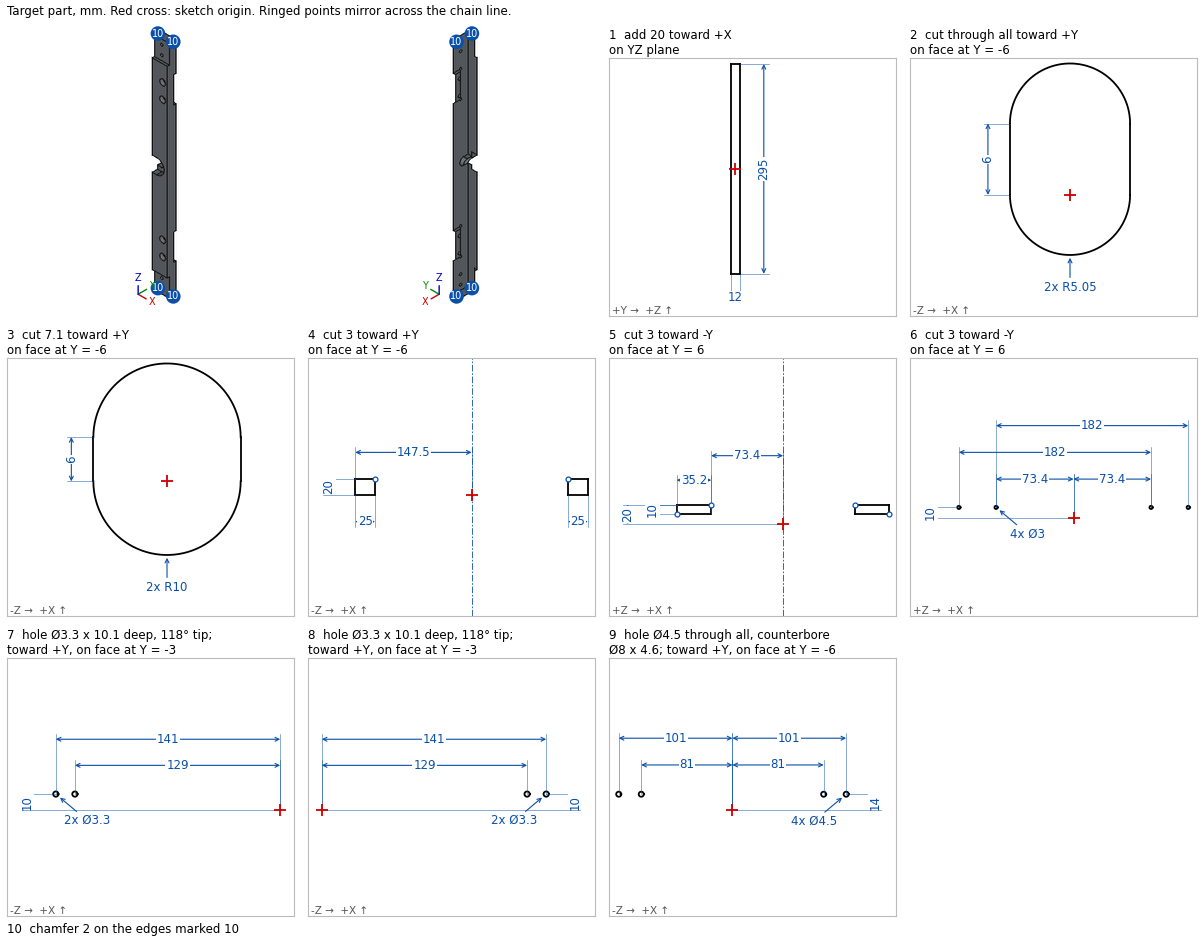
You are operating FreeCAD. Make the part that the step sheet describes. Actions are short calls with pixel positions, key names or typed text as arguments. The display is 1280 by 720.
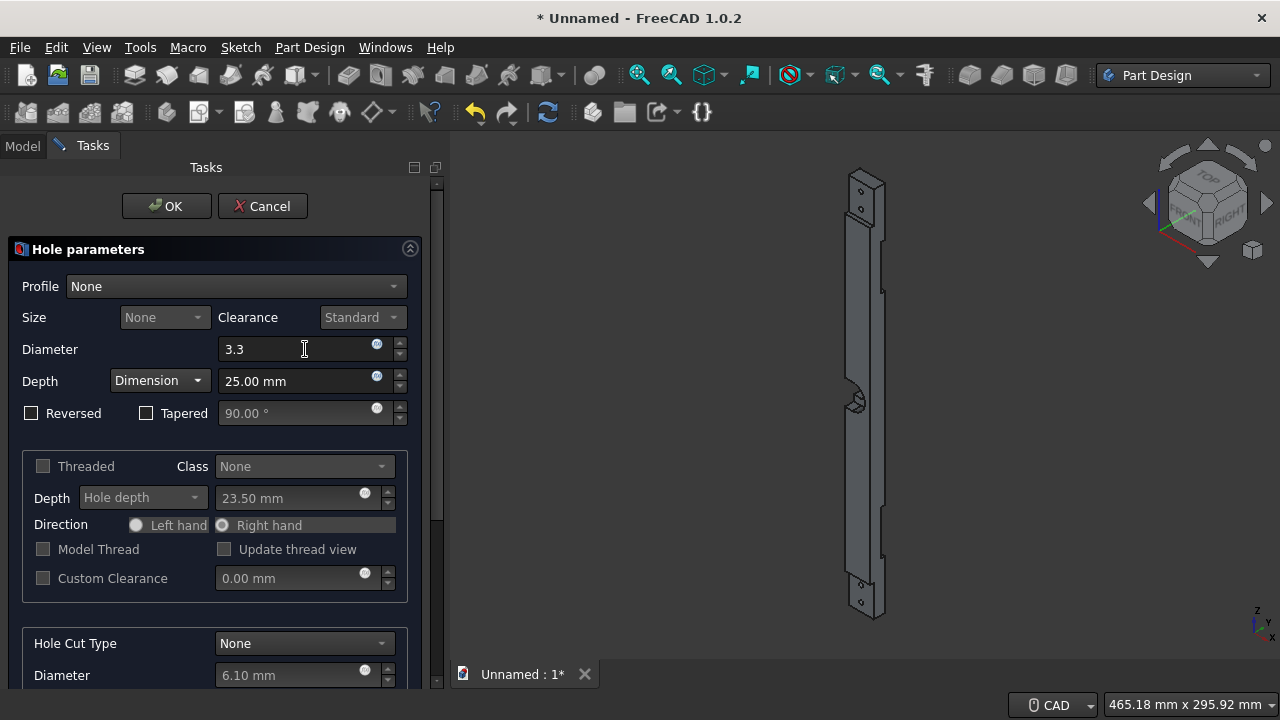
triple_click(305, 381)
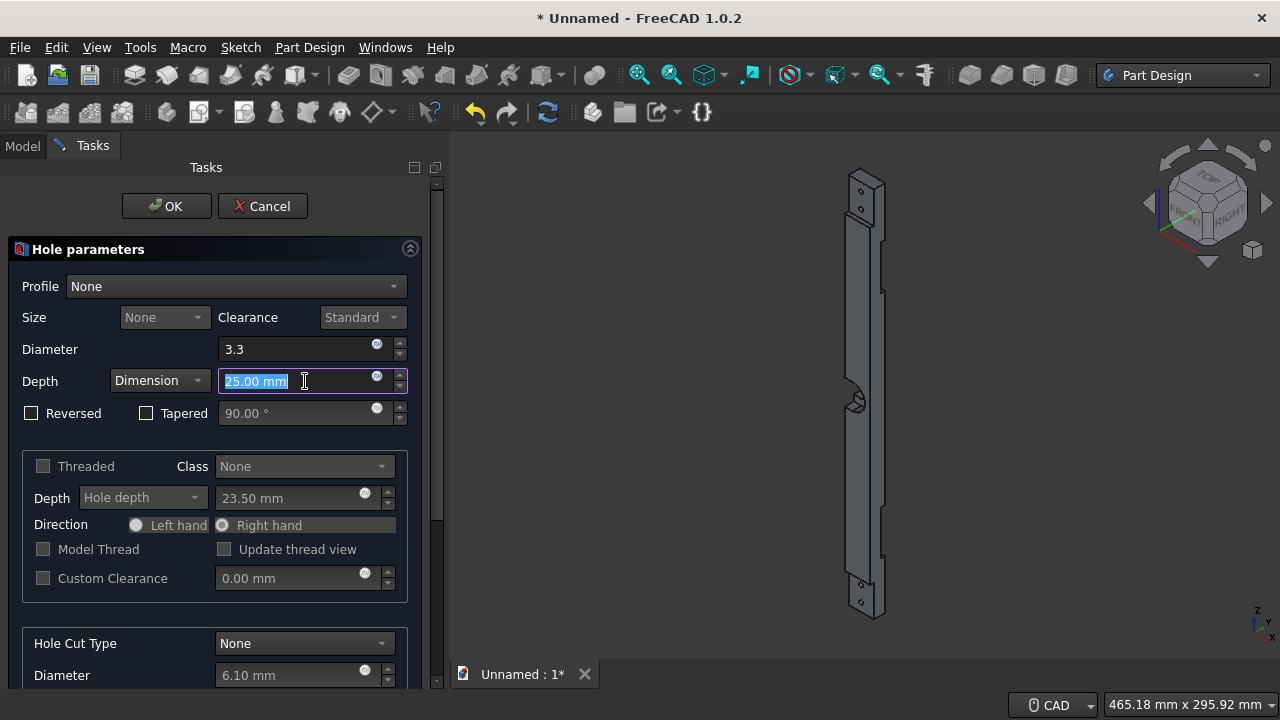
text(10.1)
key(Tab)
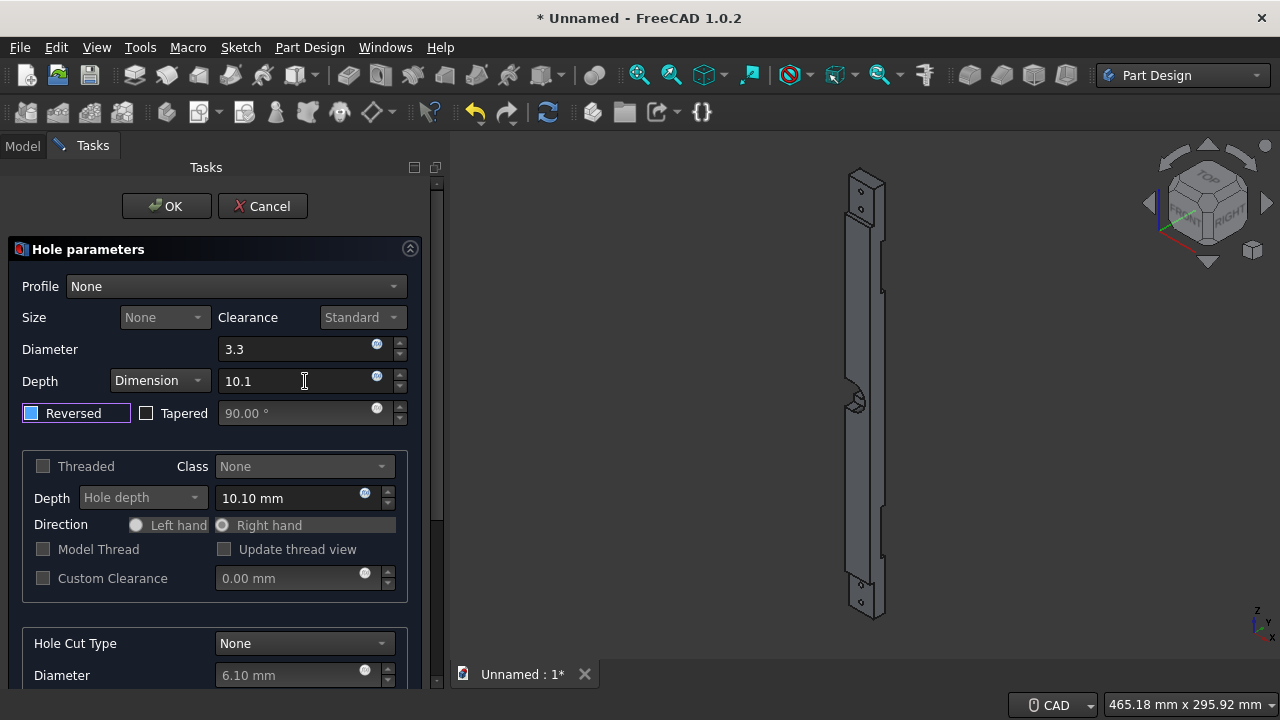
click(167, 206)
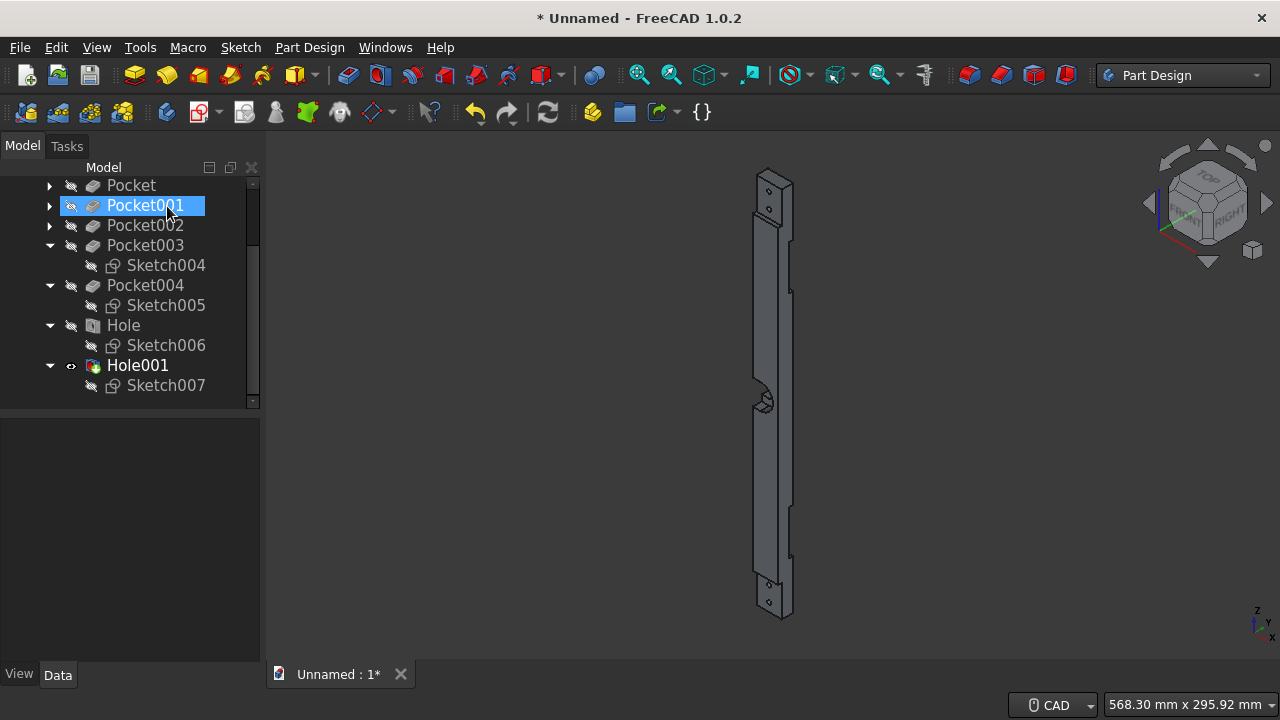
click(765, 347)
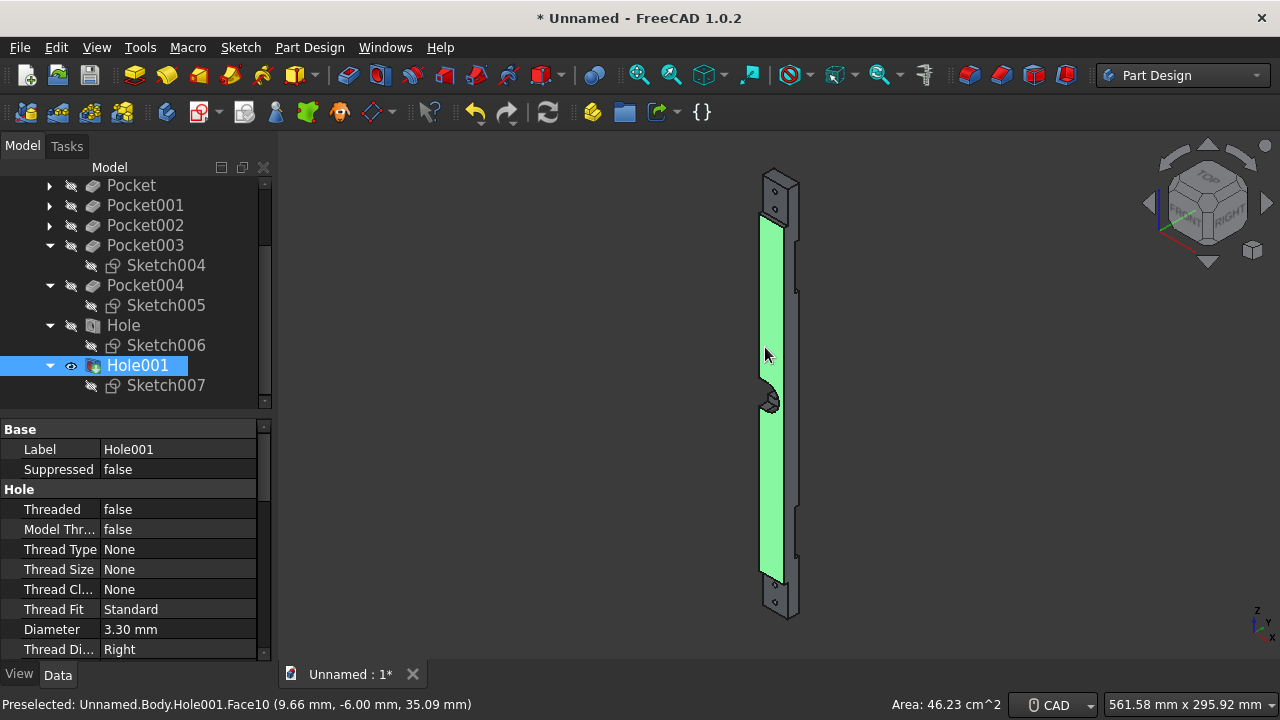
click(200, 112)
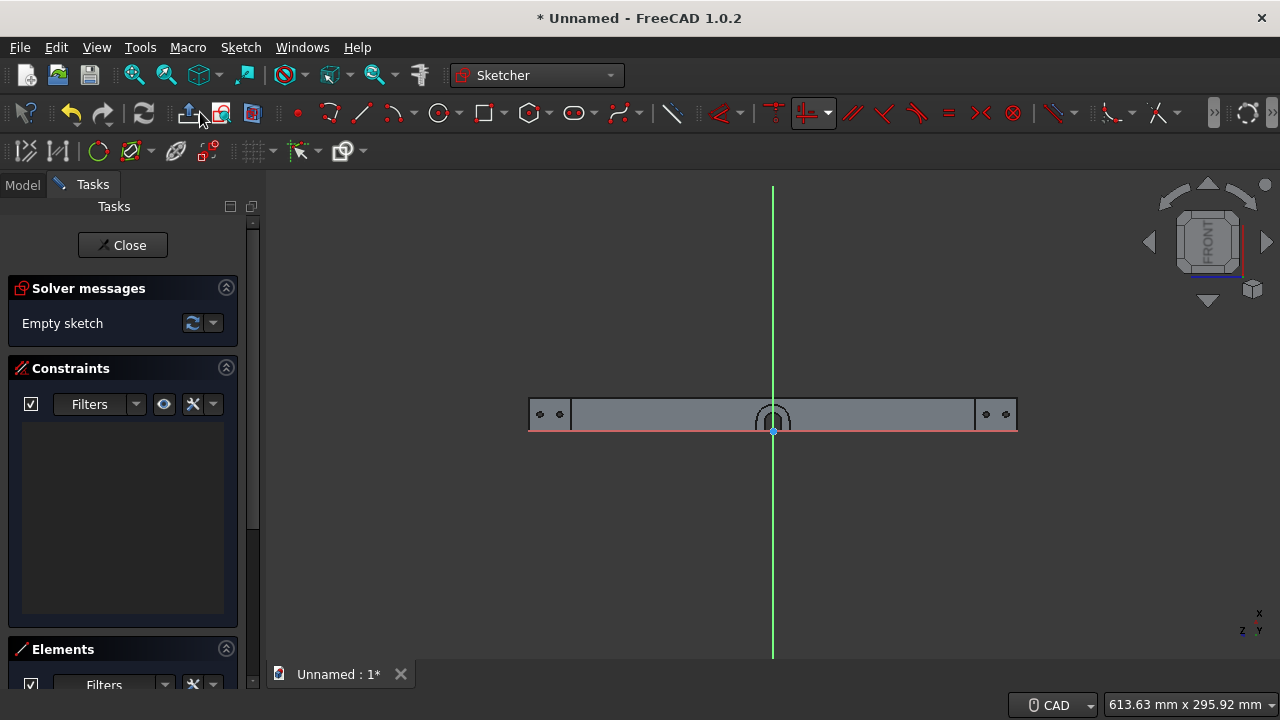
scroll(856, 421, up, 3)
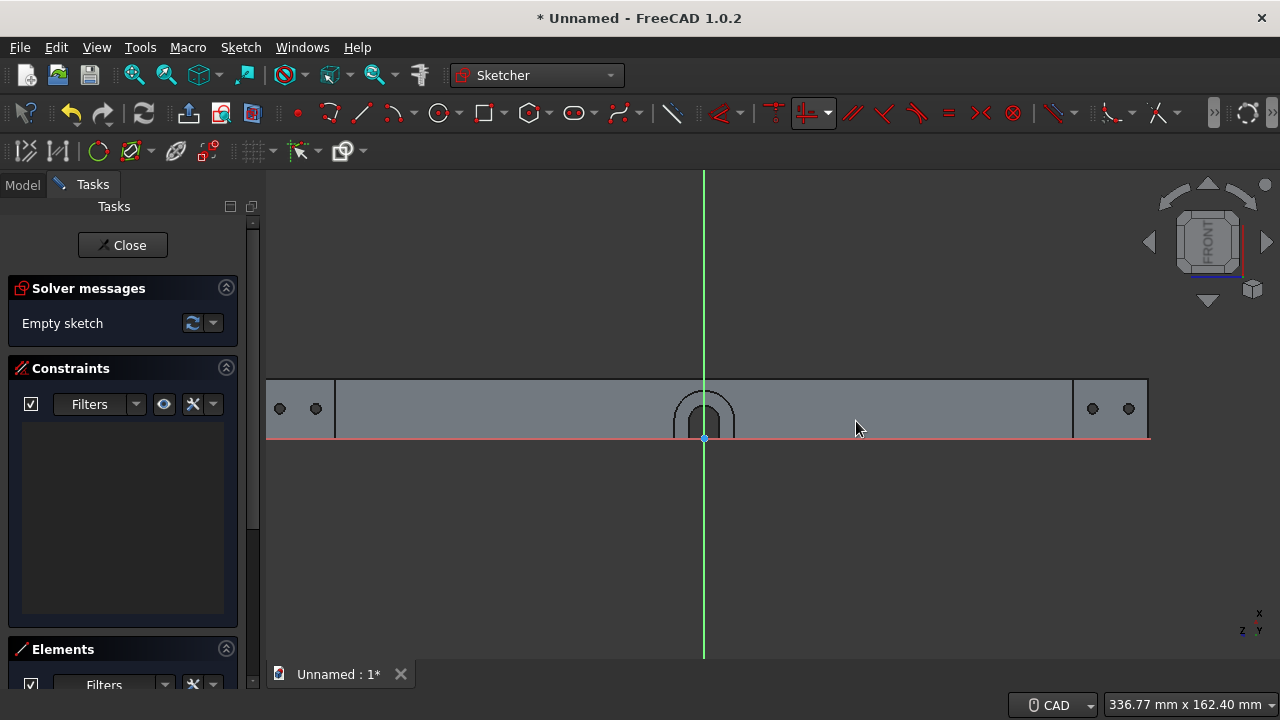
click(440, 114)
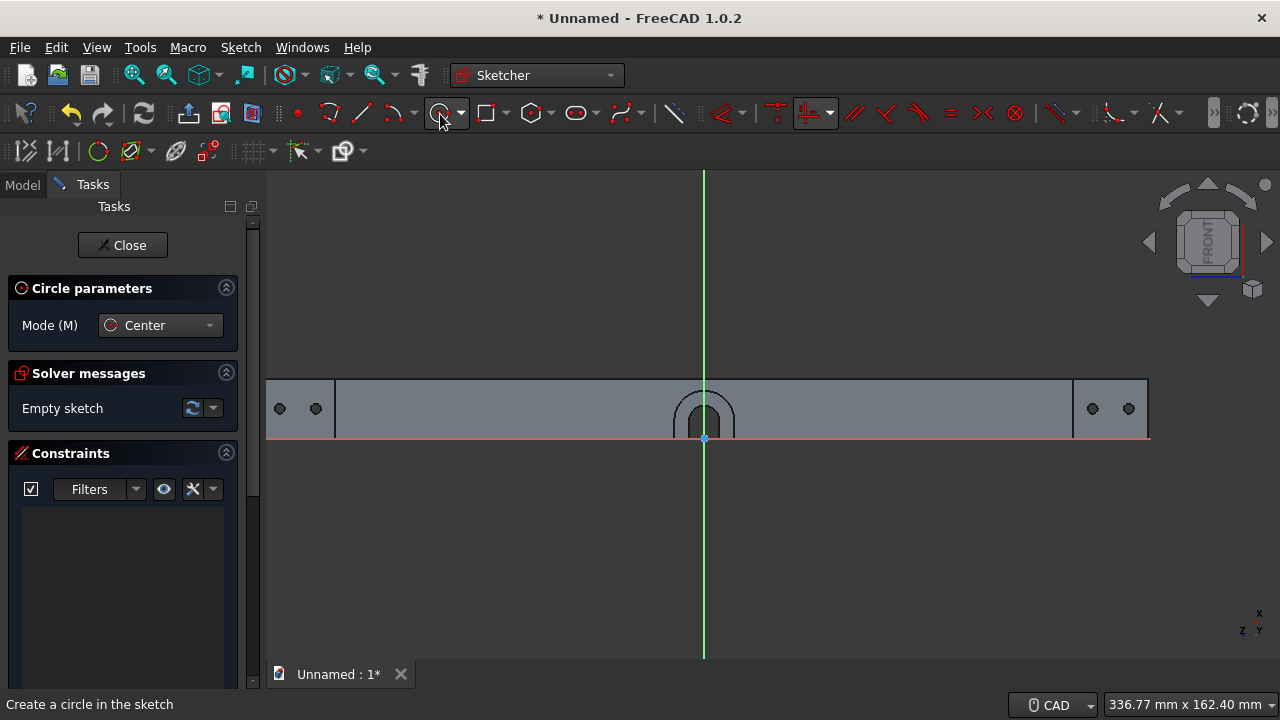
scroll(1008, 397, up, 7)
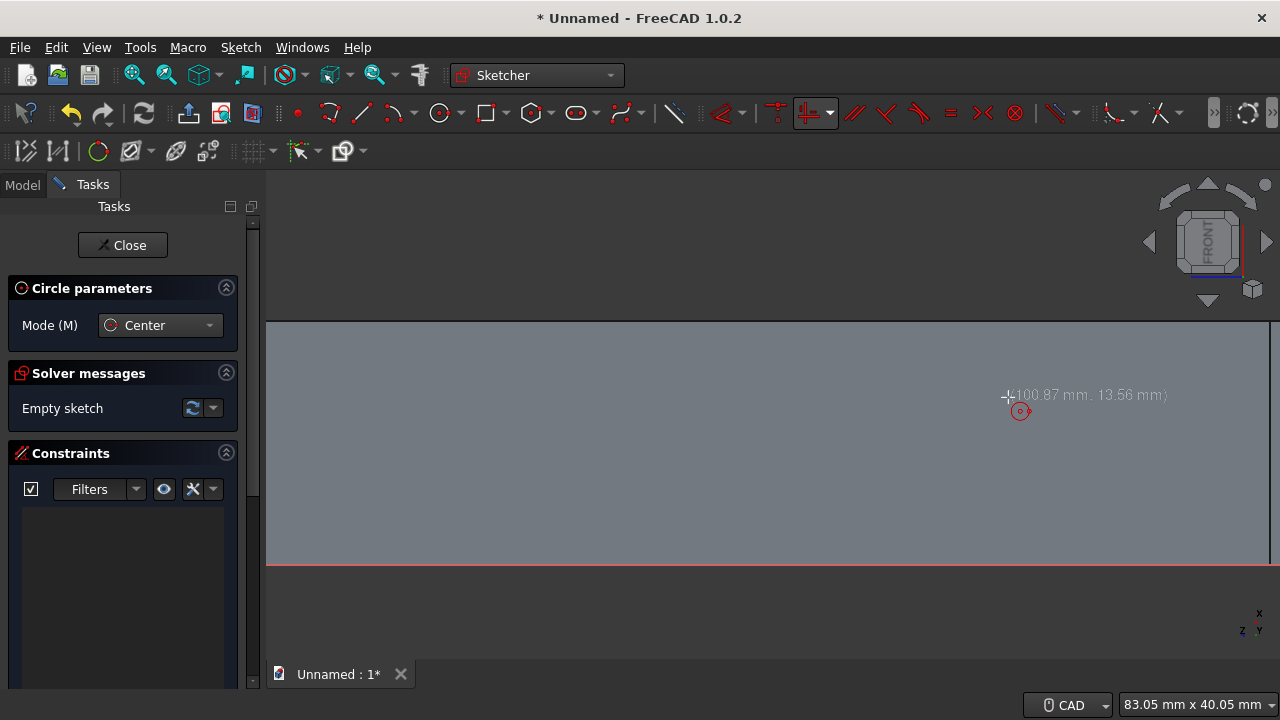
scroll(1009, 398, down, 7)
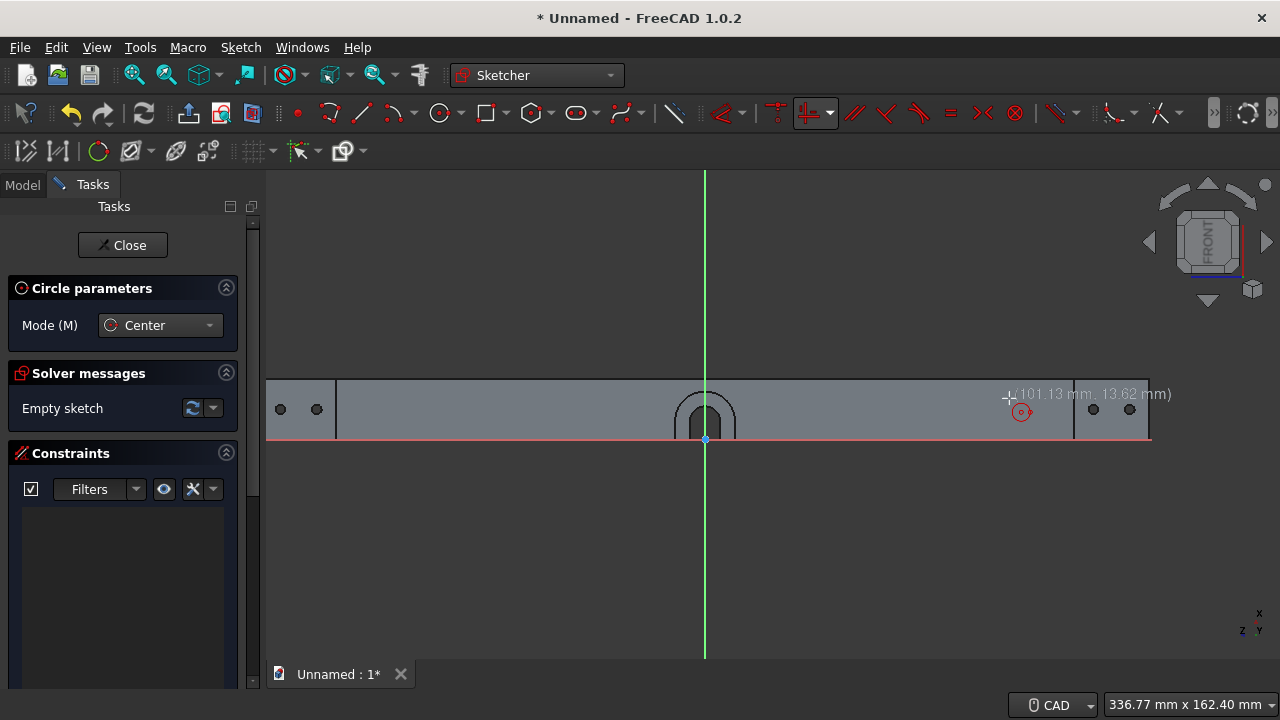
click(1009, 397)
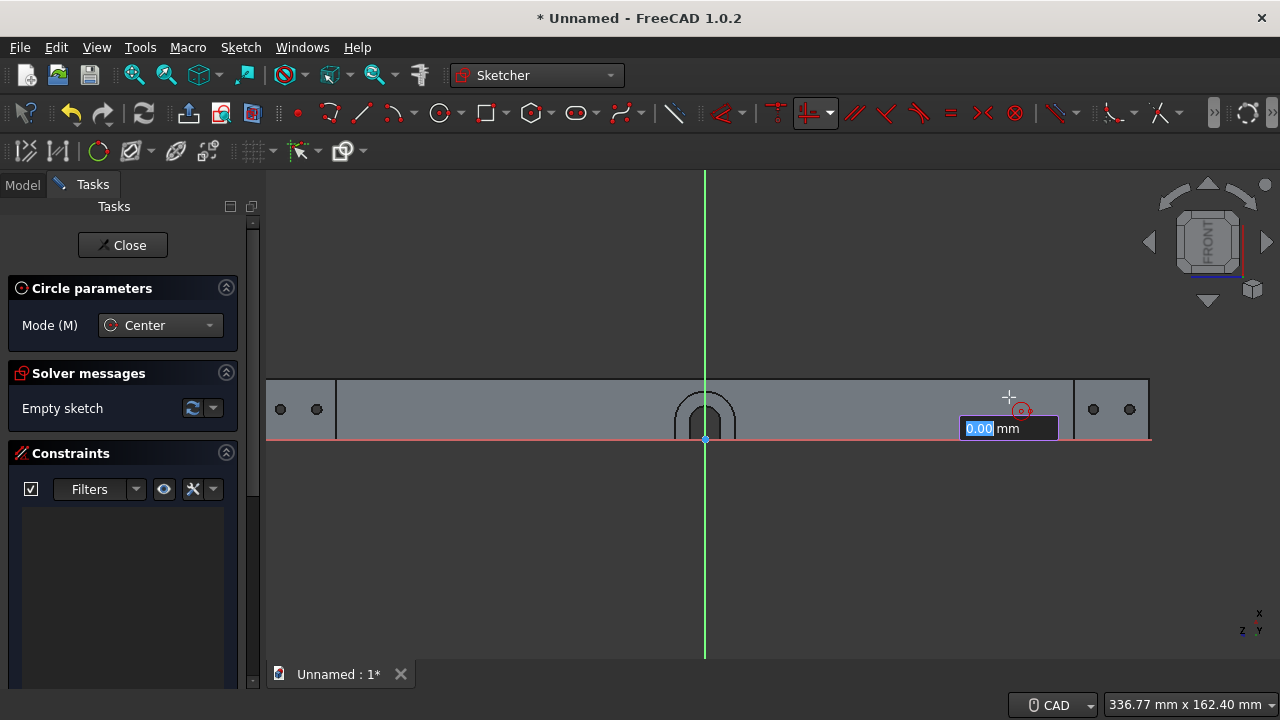
scroll(1014, 393, up, 5)